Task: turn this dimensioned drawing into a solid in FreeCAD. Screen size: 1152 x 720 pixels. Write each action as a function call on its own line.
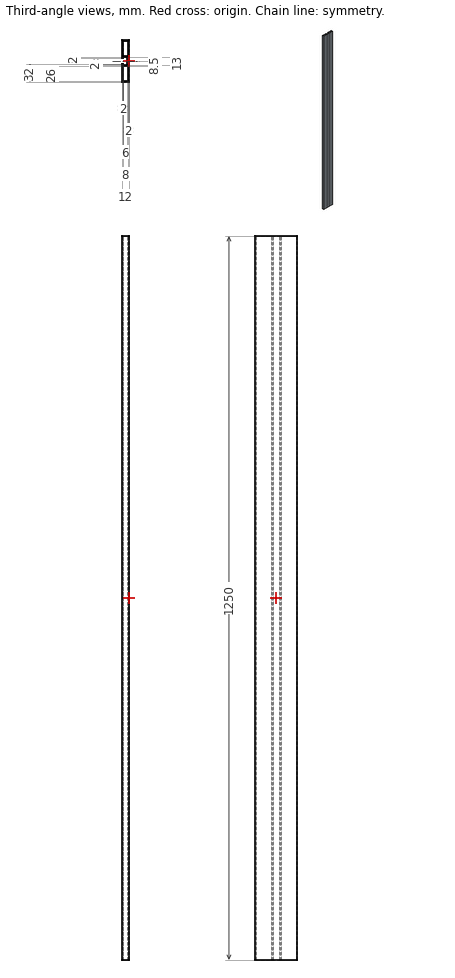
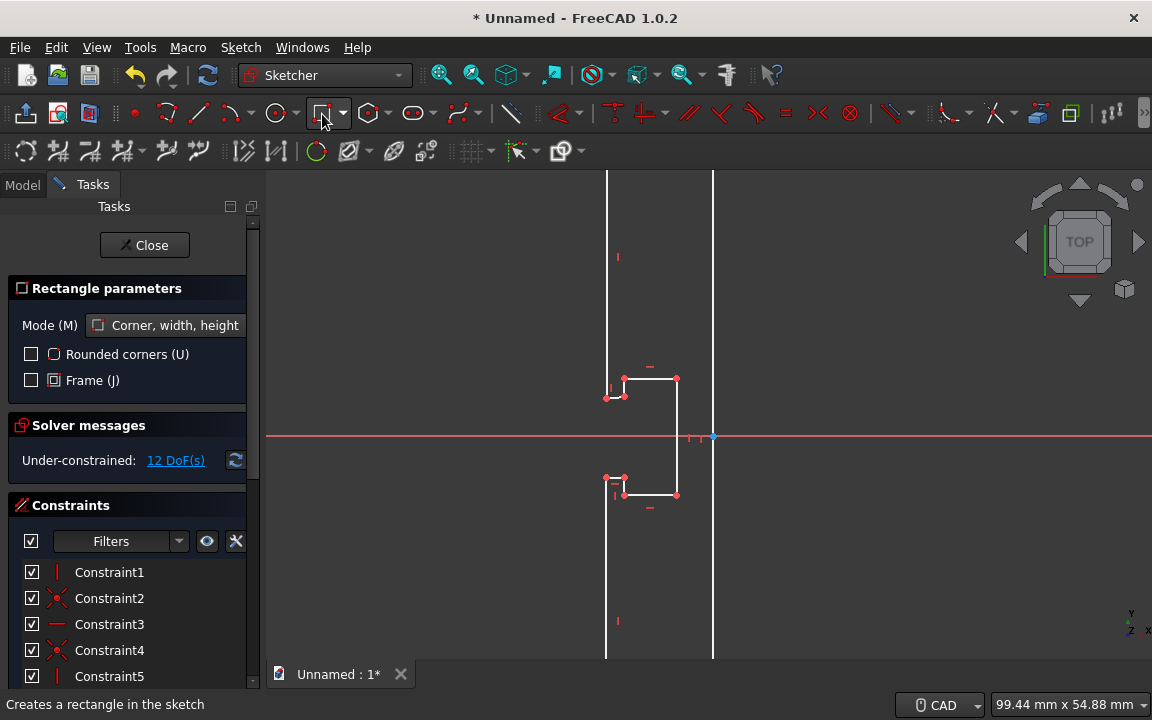
click(624, 512)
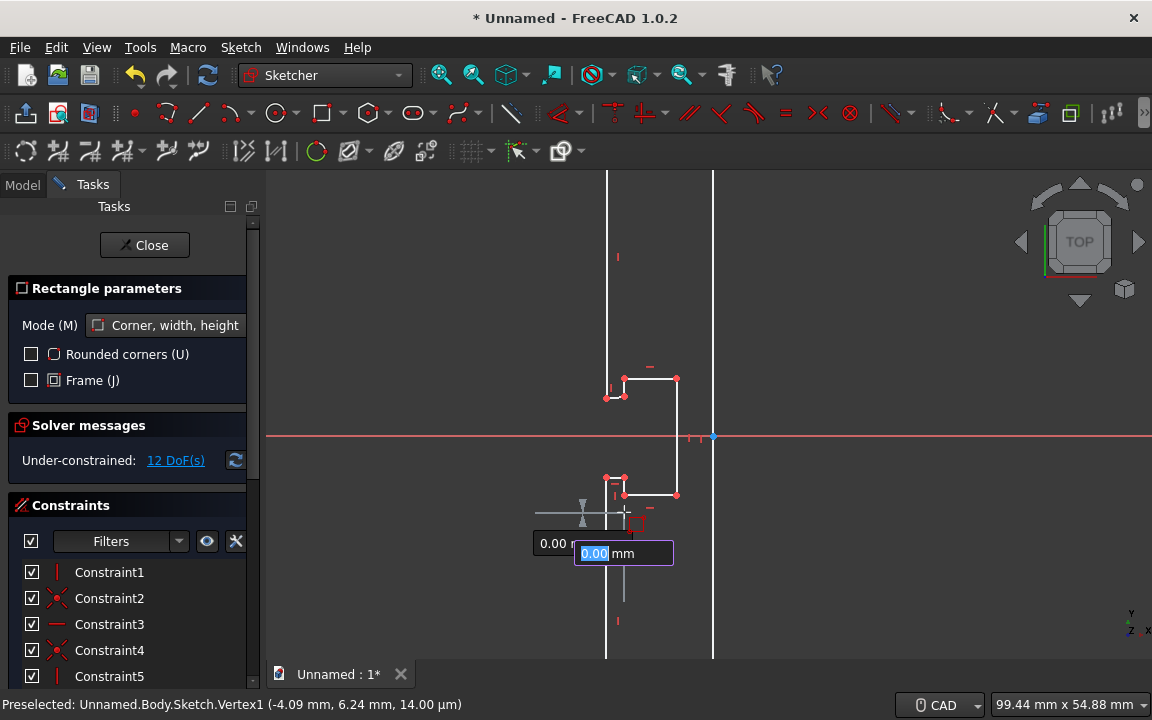
scroll(625, 397, down, 4)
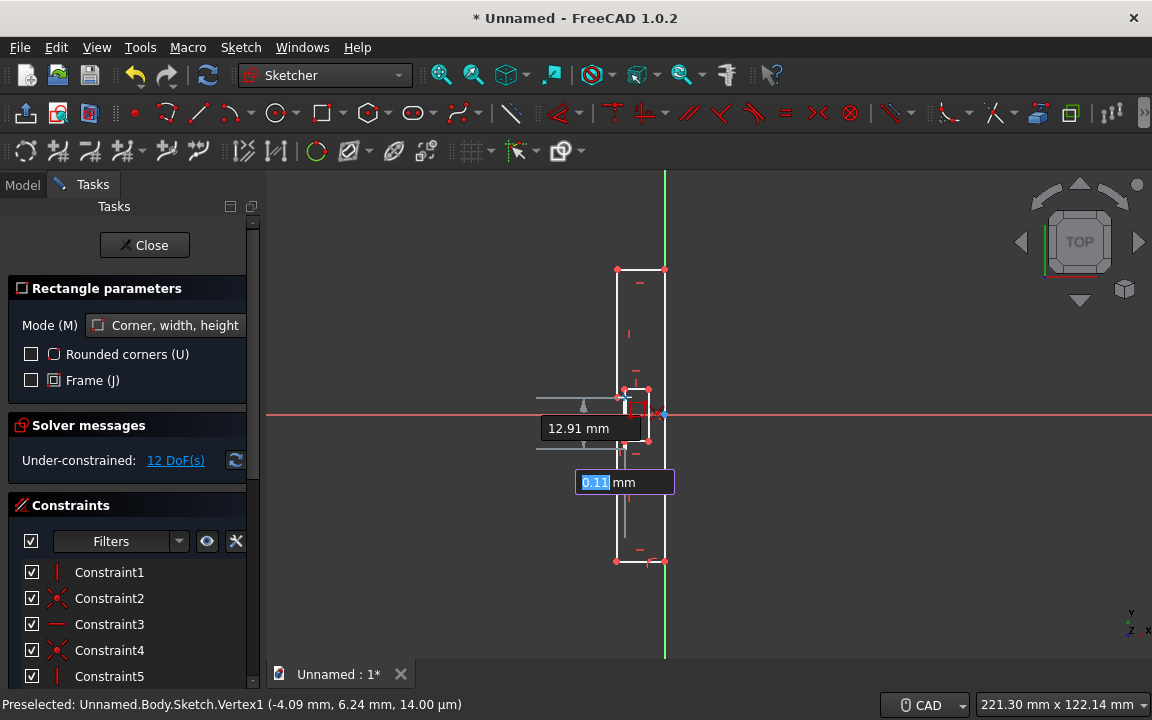
scroll(657, 553, up, 4)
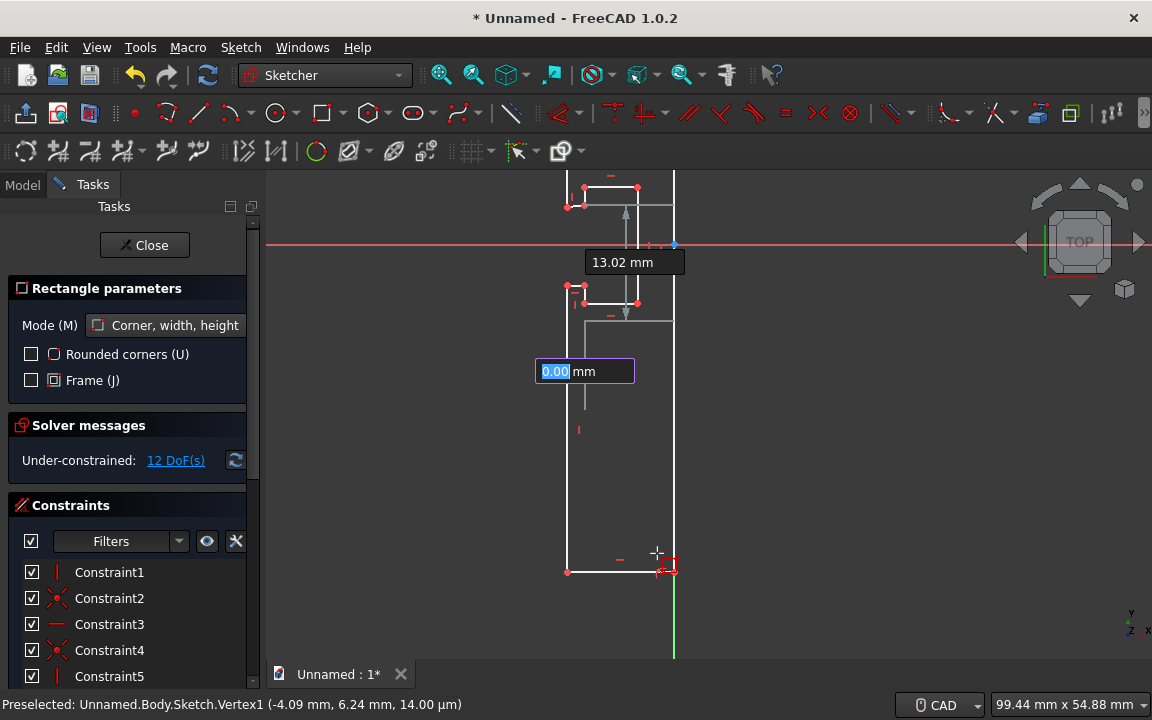
click(656, 552)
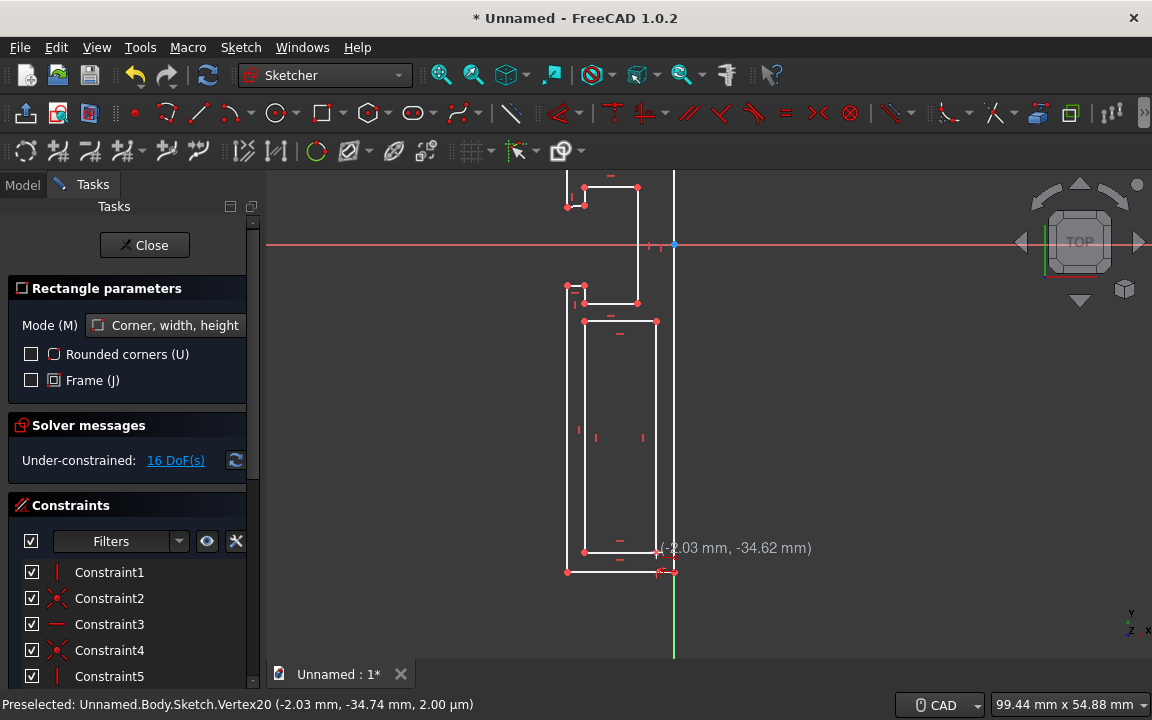
scroll(657, 553, down, 4)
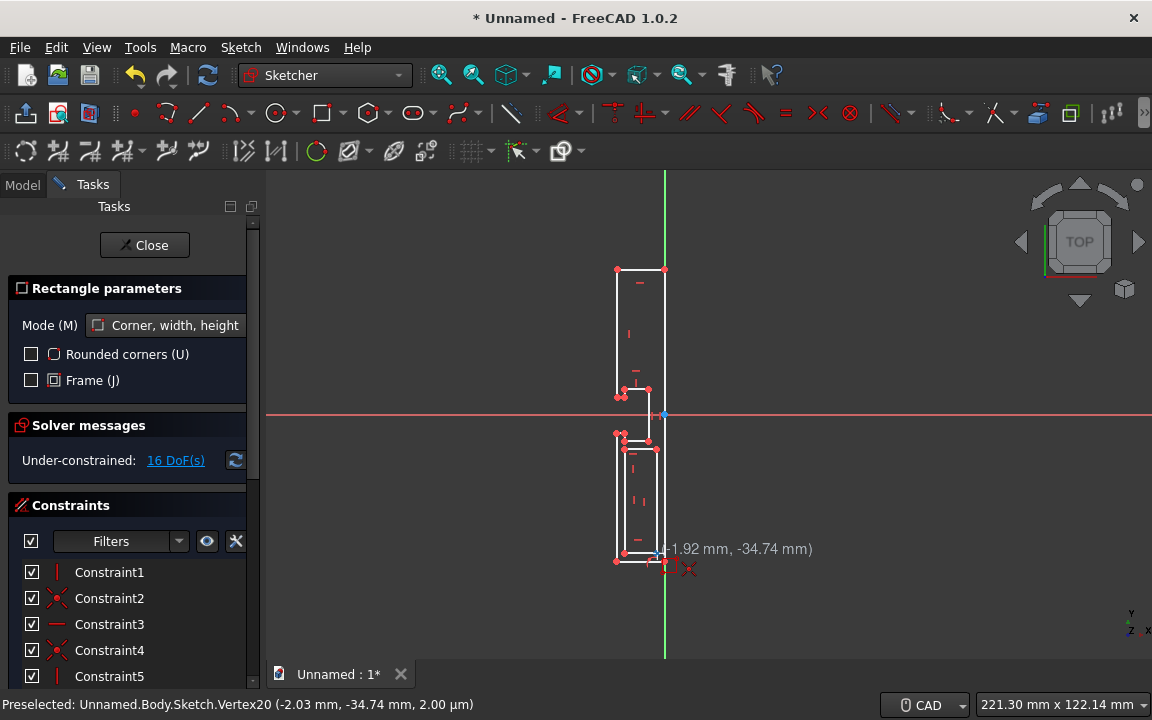
scroll(625, 277, up, 4)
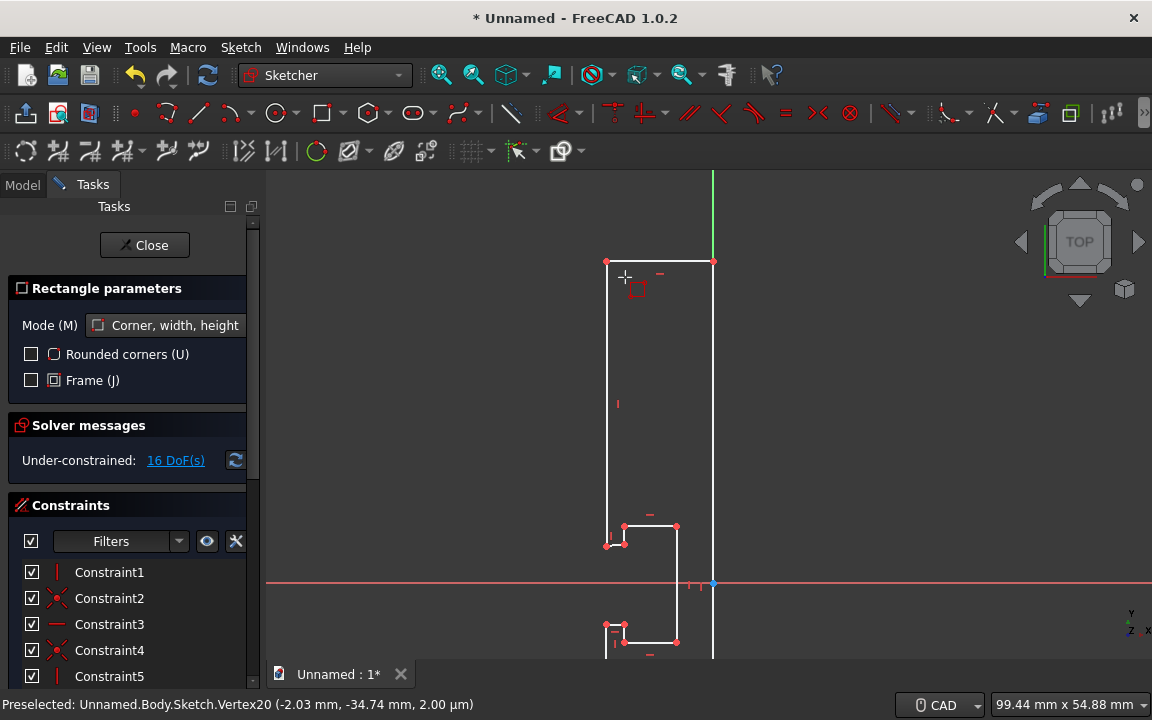
click(624, 276)
click(696, 508)
key(Escape)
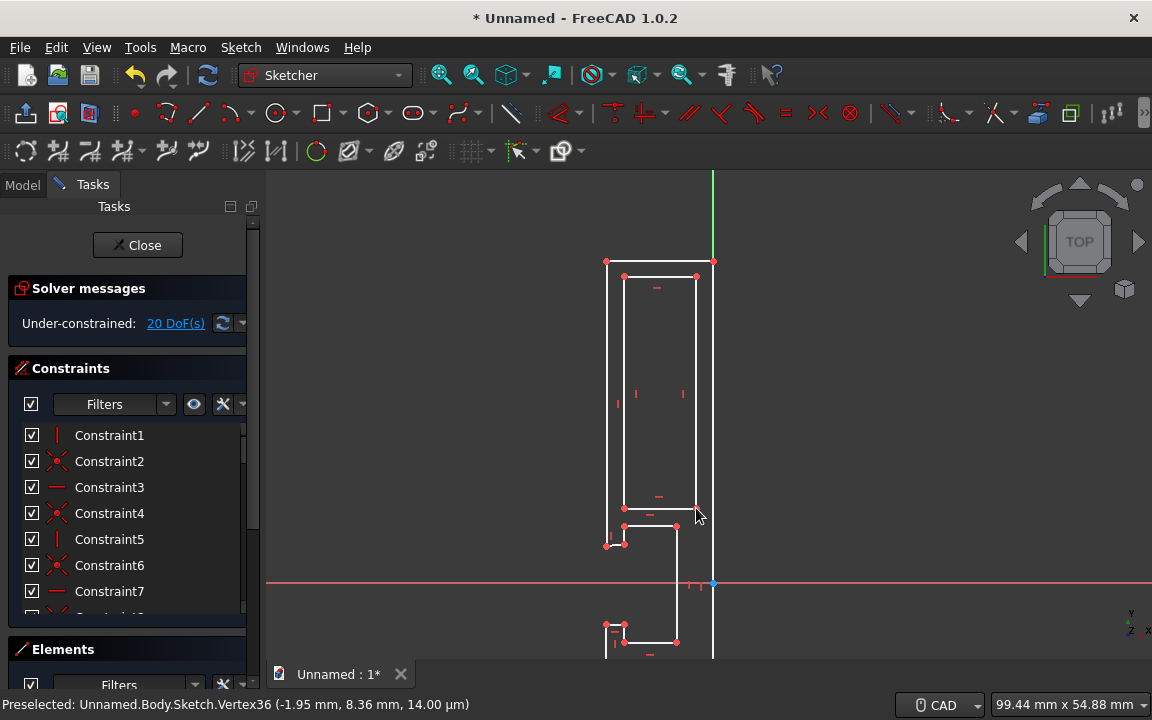
scroll(615, 545, up, 3)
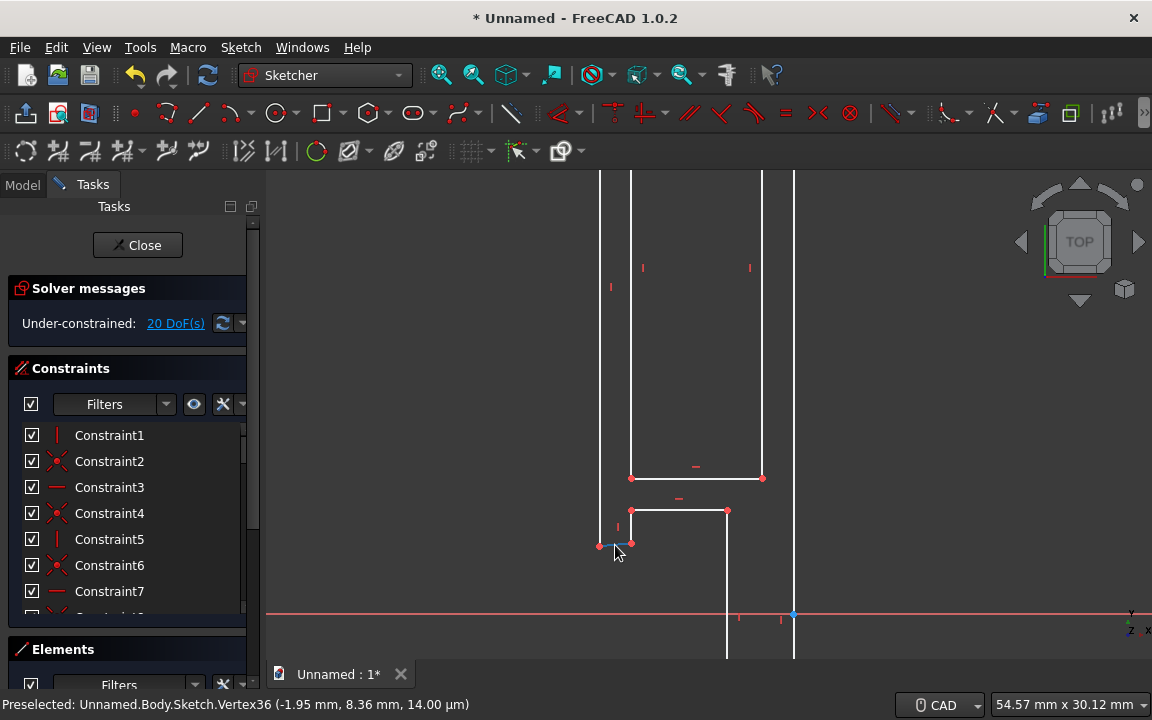
click(615, 545)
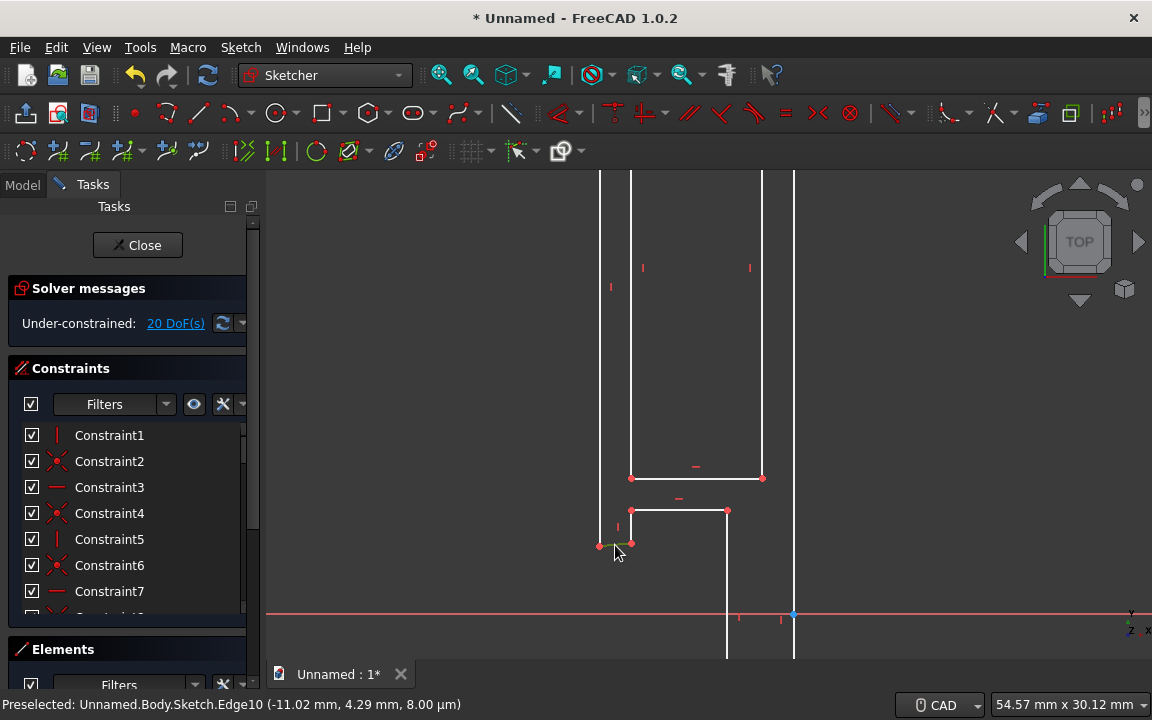
click(668, 114)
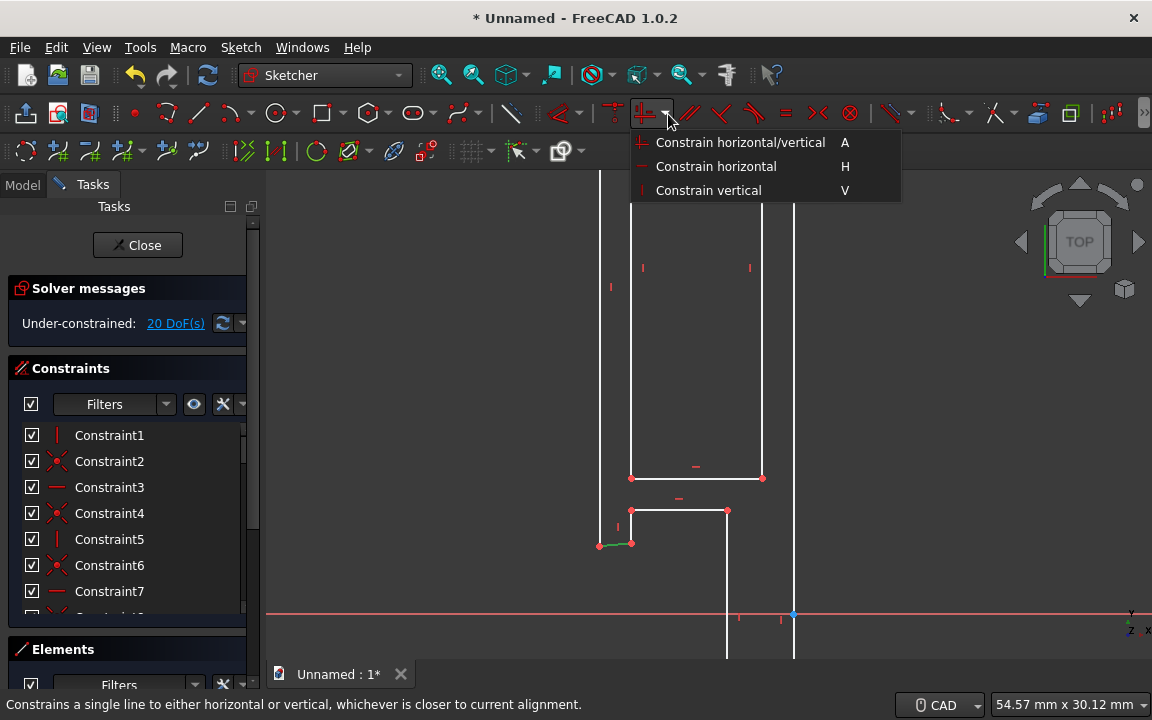
click(766, 166)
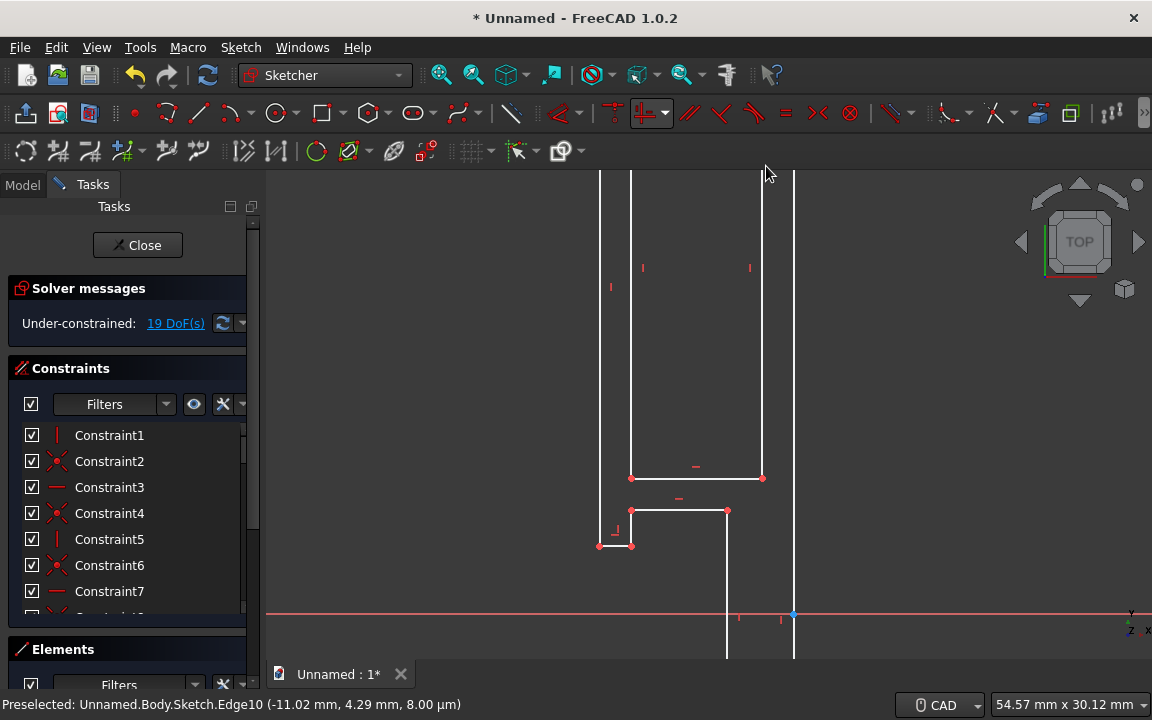
scroll(622, 349, down, 7)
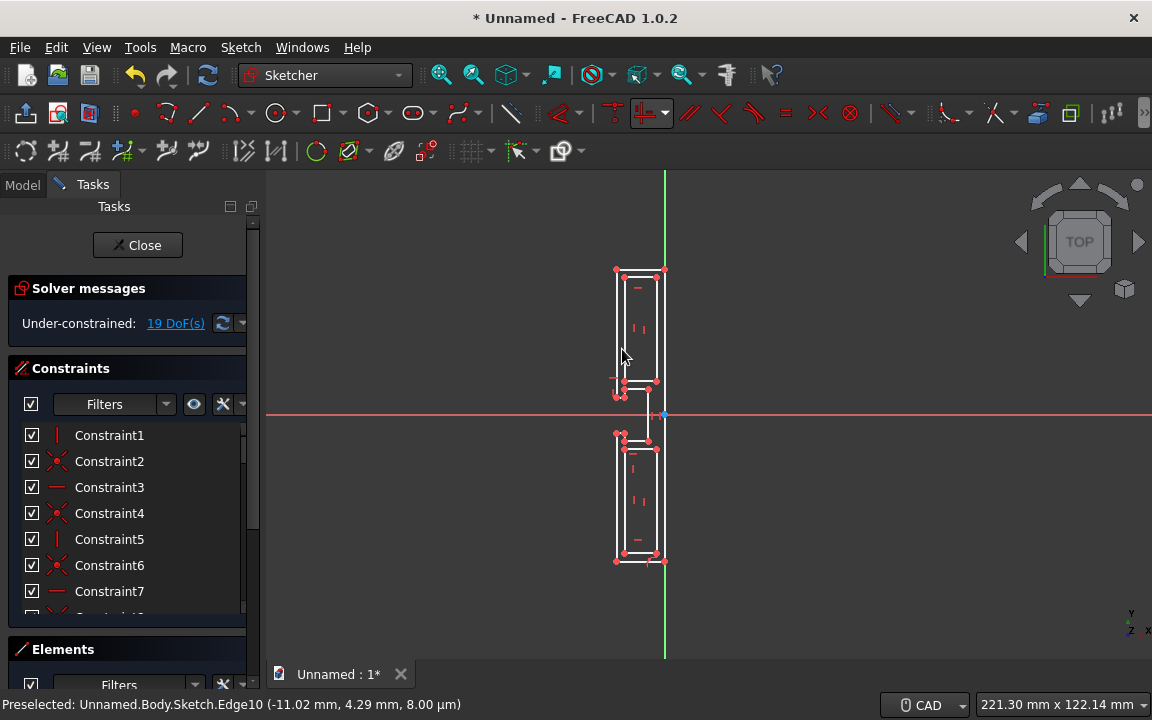
click(617, 562)